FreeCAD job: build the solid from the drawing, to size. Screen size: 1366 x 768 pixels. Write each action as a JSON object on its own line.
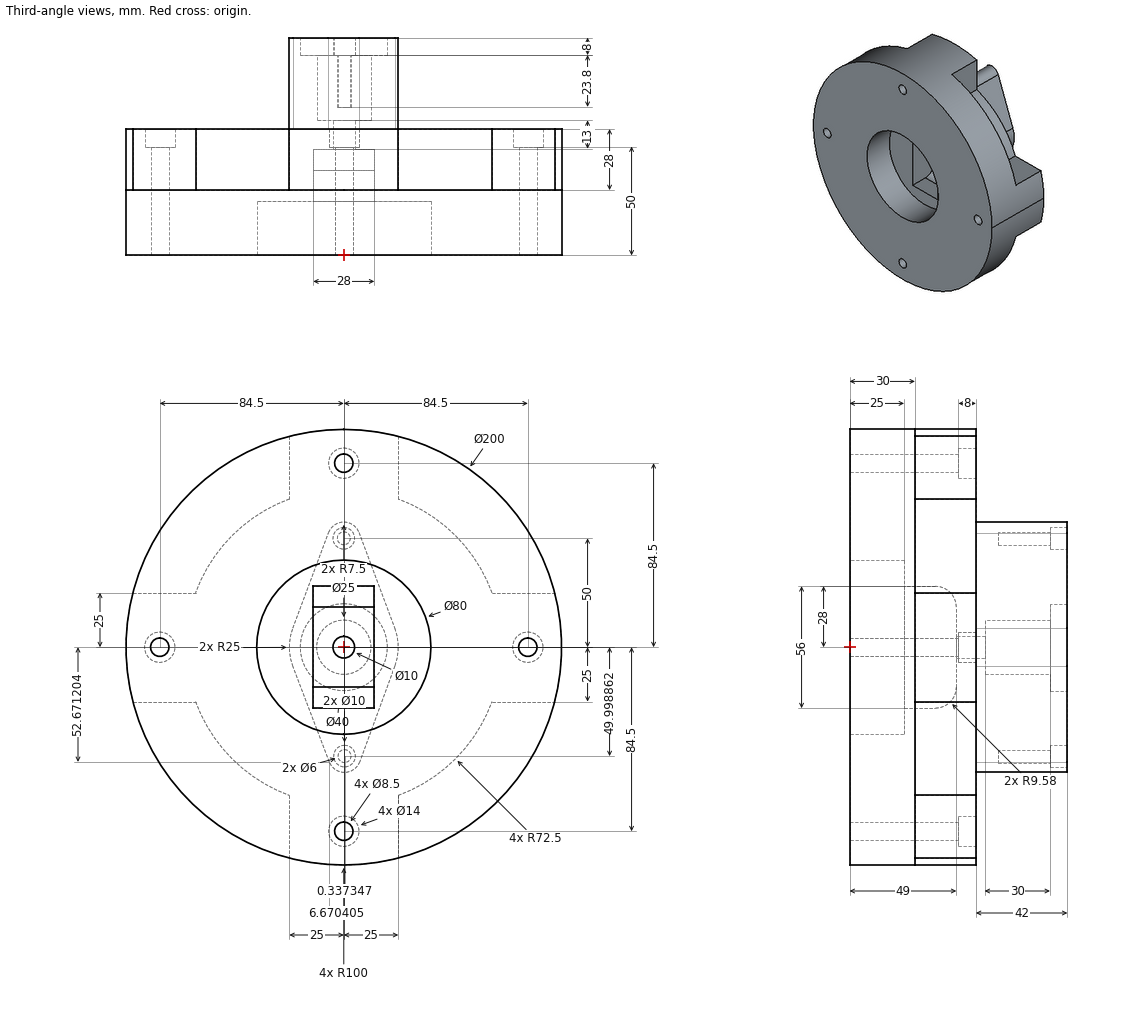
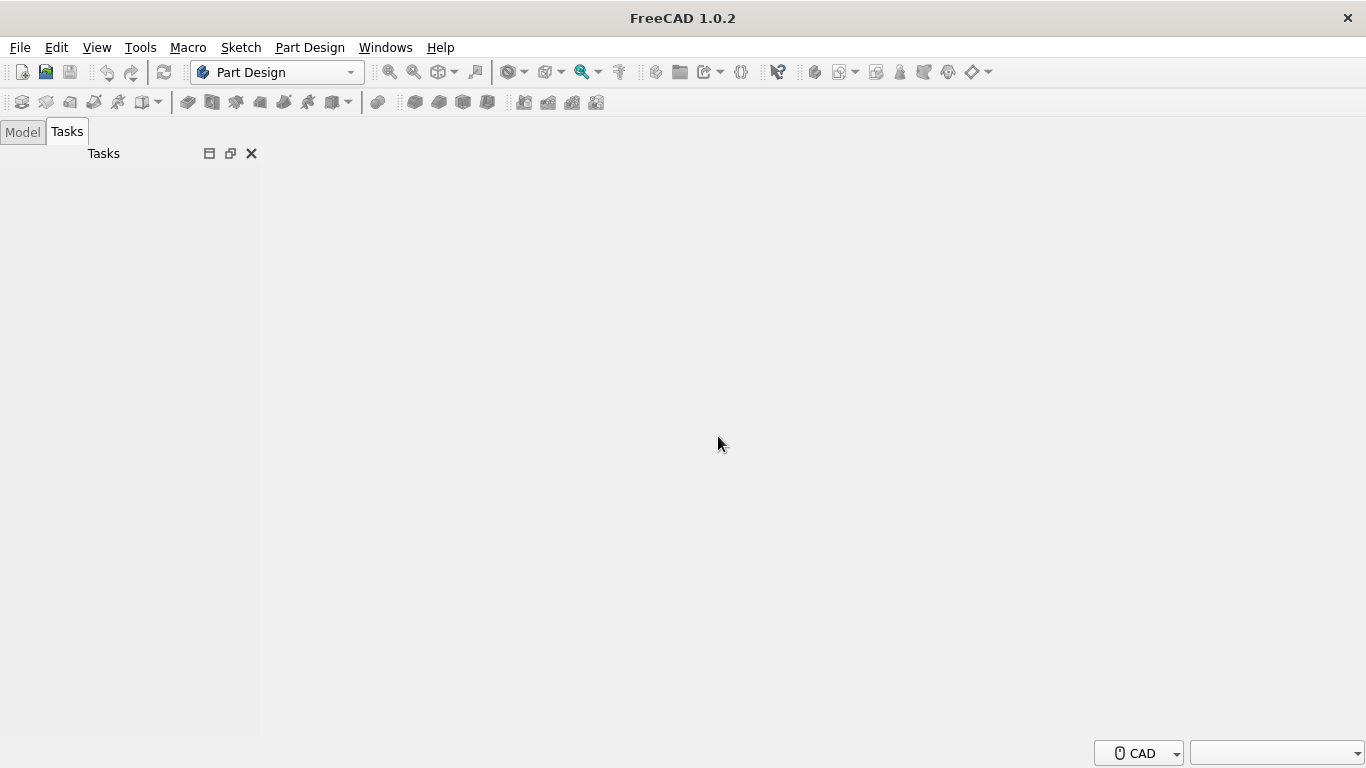
{"action": "key", "text": "ctrl+n"}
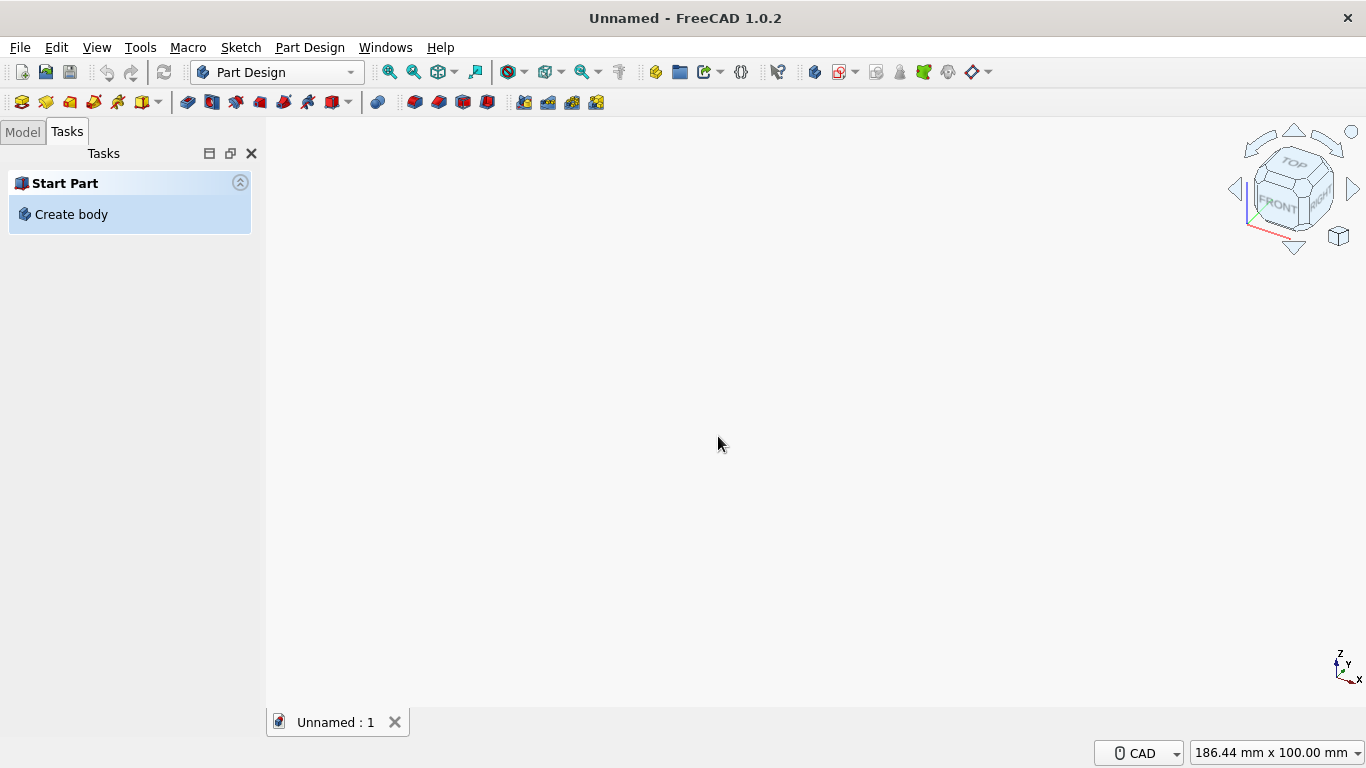
{"action": "left_click", "coordinate": [840, 72]}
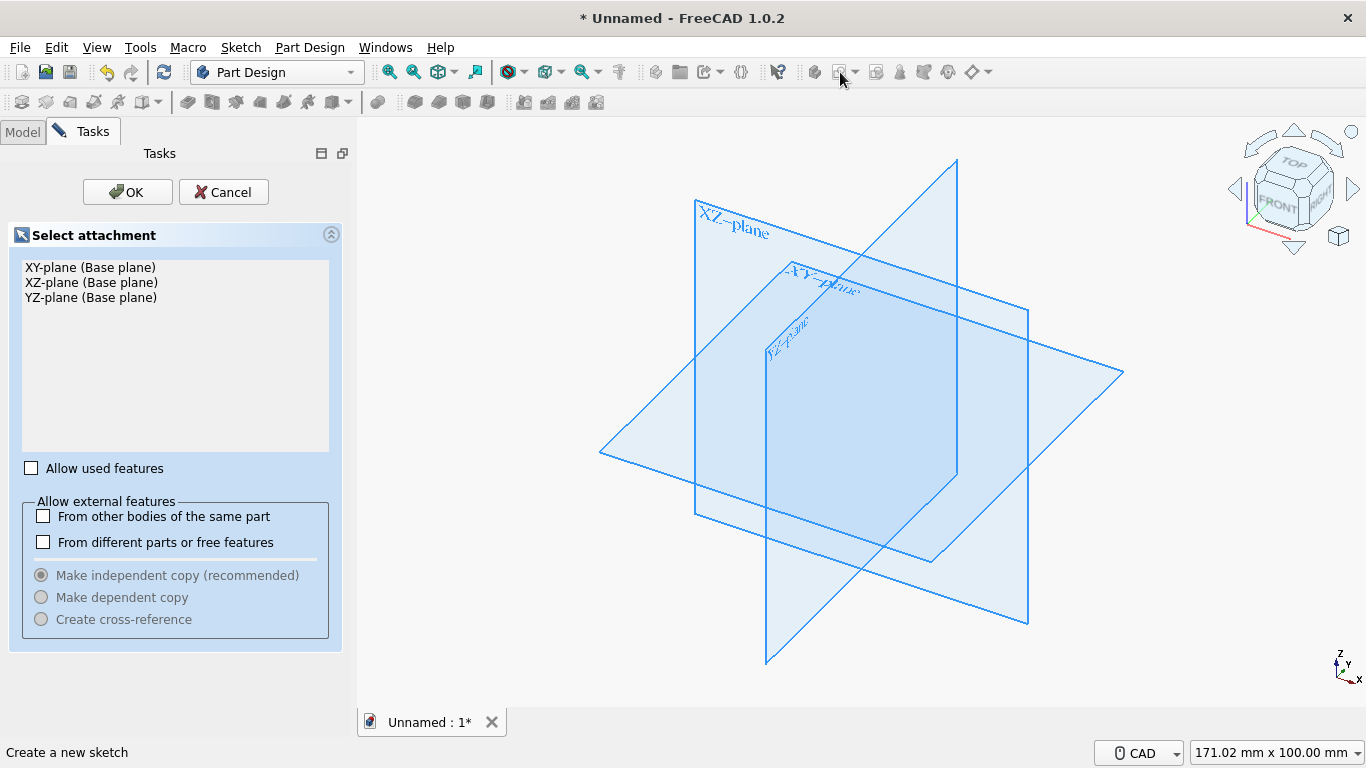
{"action": "left_click", "coordinate": [82, 282]}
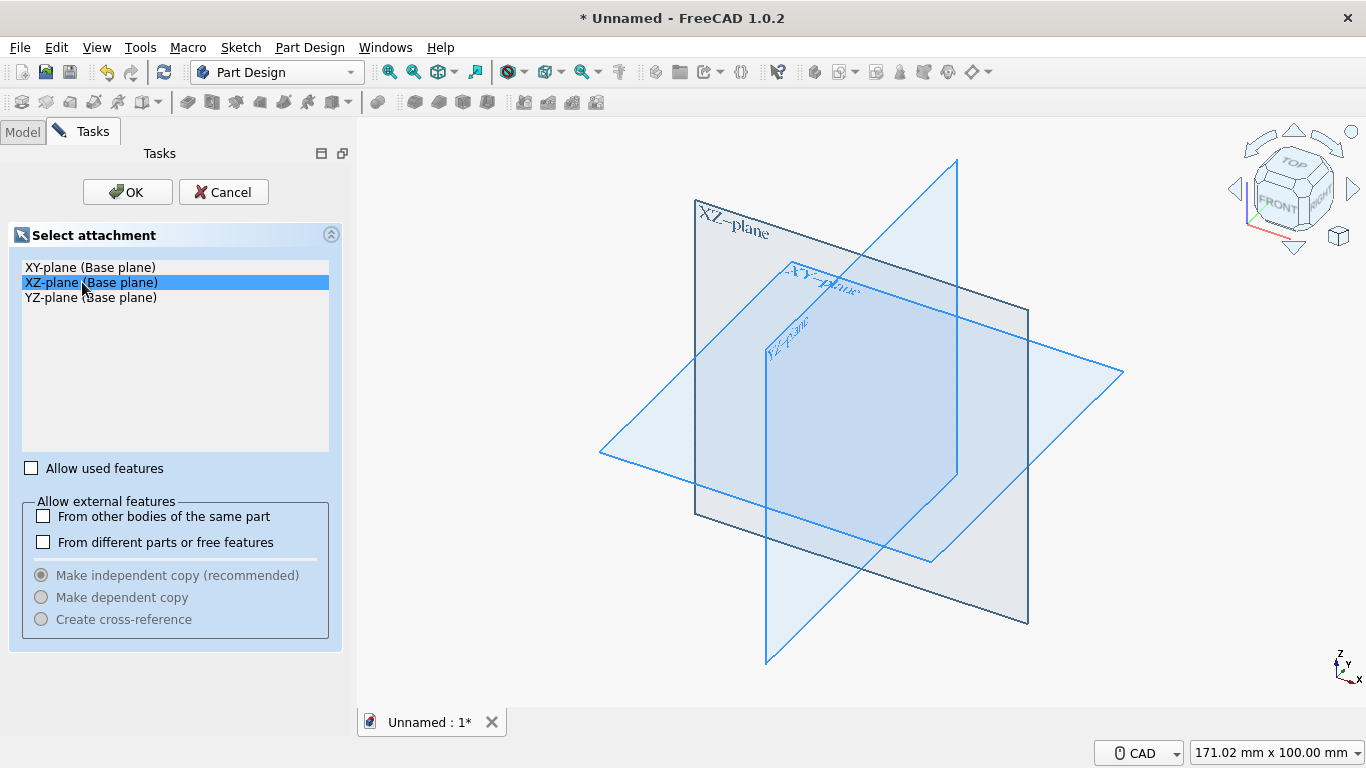
{"action": "left_click", "coordinate": [128, 192]}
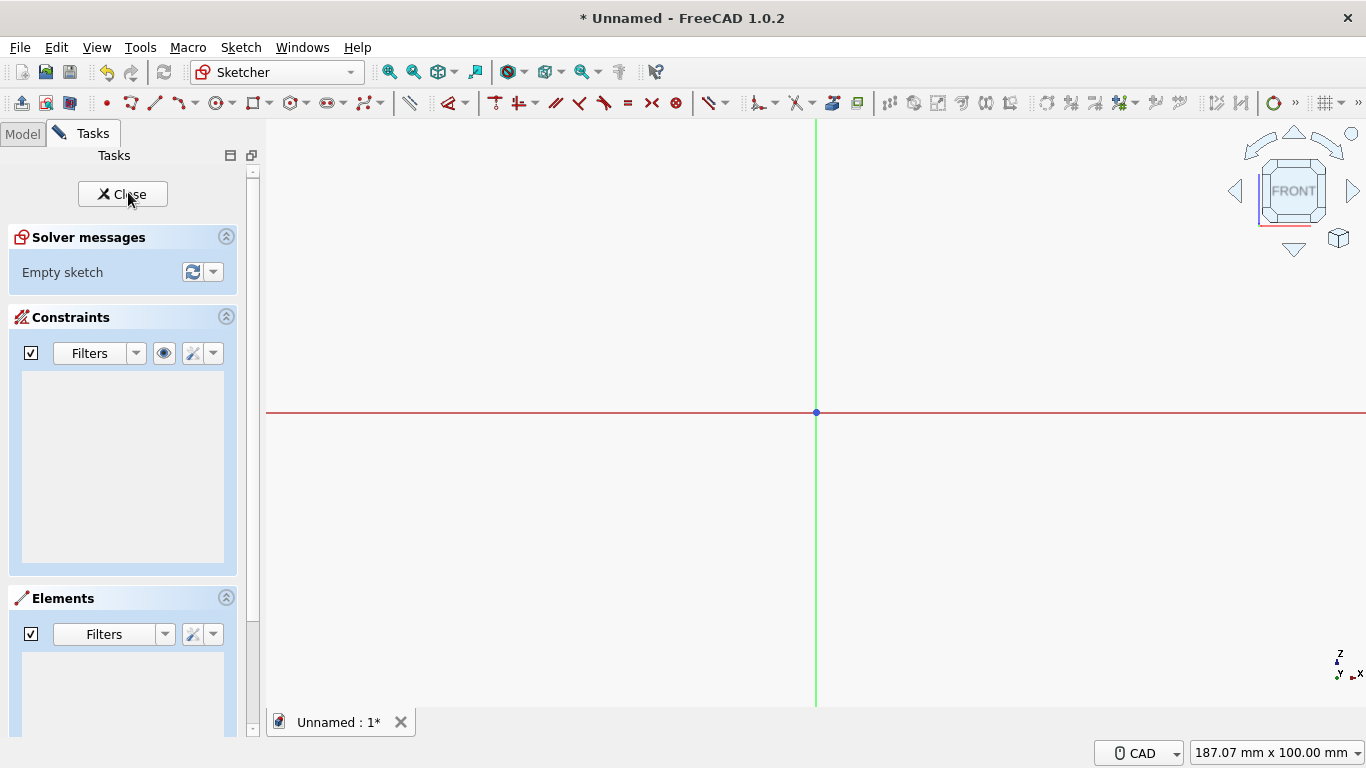
{"action": "scroll", "coordinate": [718, 413], "scroll_direction": "down", "scroll_amount": 6}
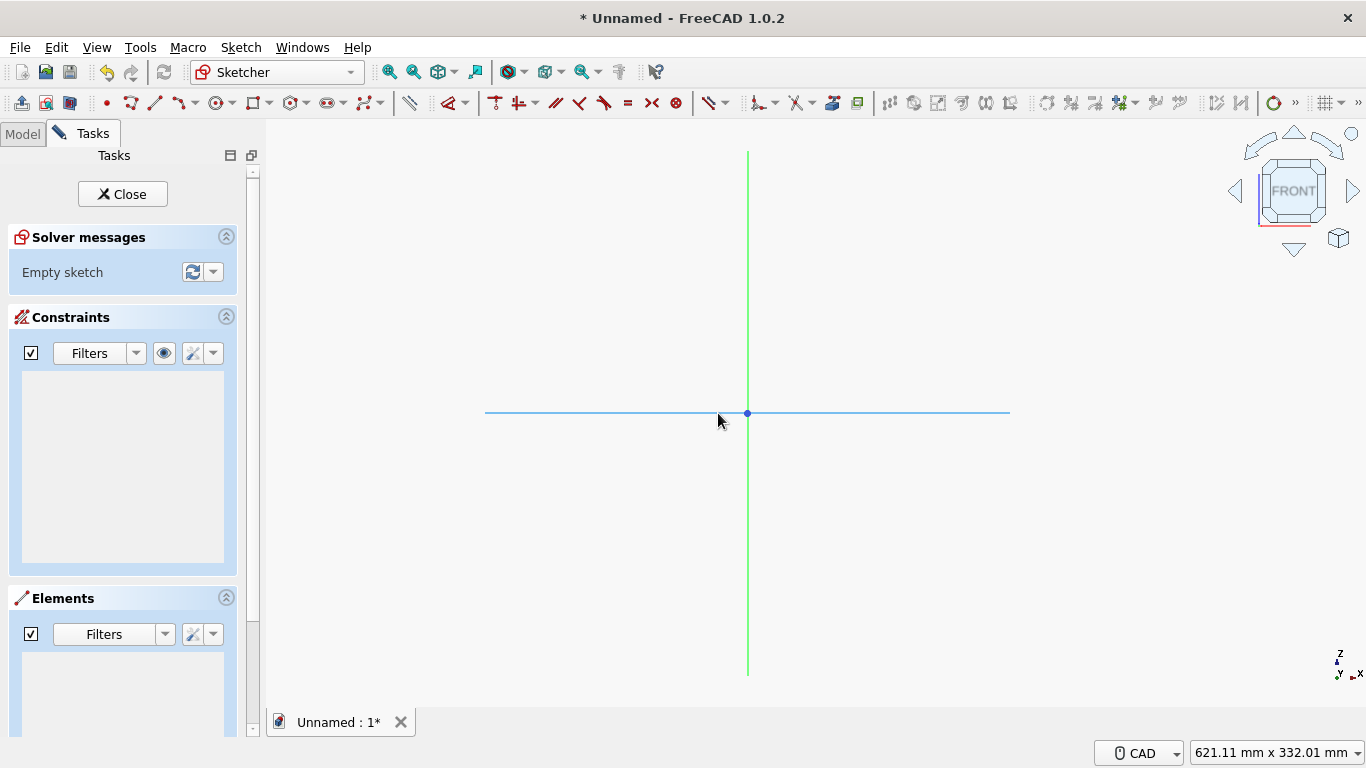
{"action": "key", "text": "g c"}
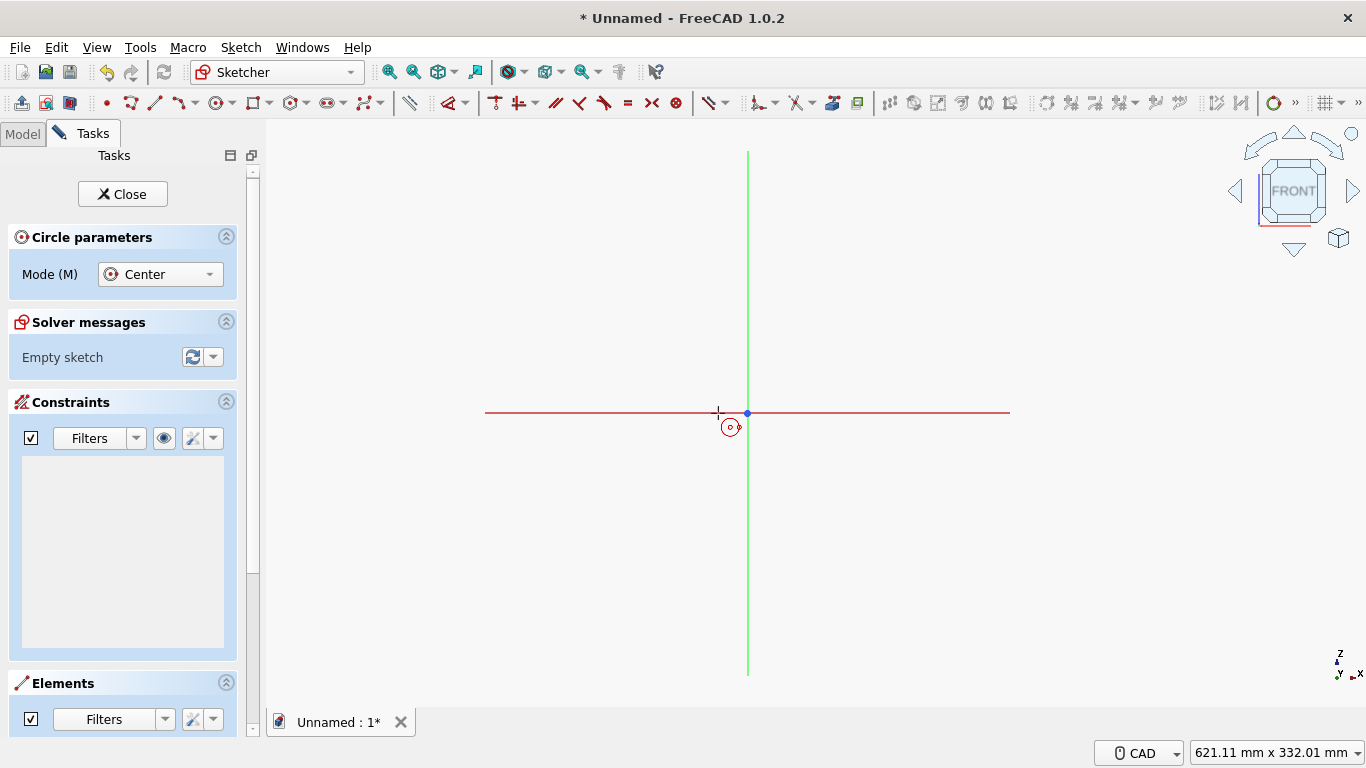
{"action": "left_click", "coordinate": [748, 413]}
{"action": "left_click", "coordinate": [873, 288]}
{"action": "key", "text": "Escape"}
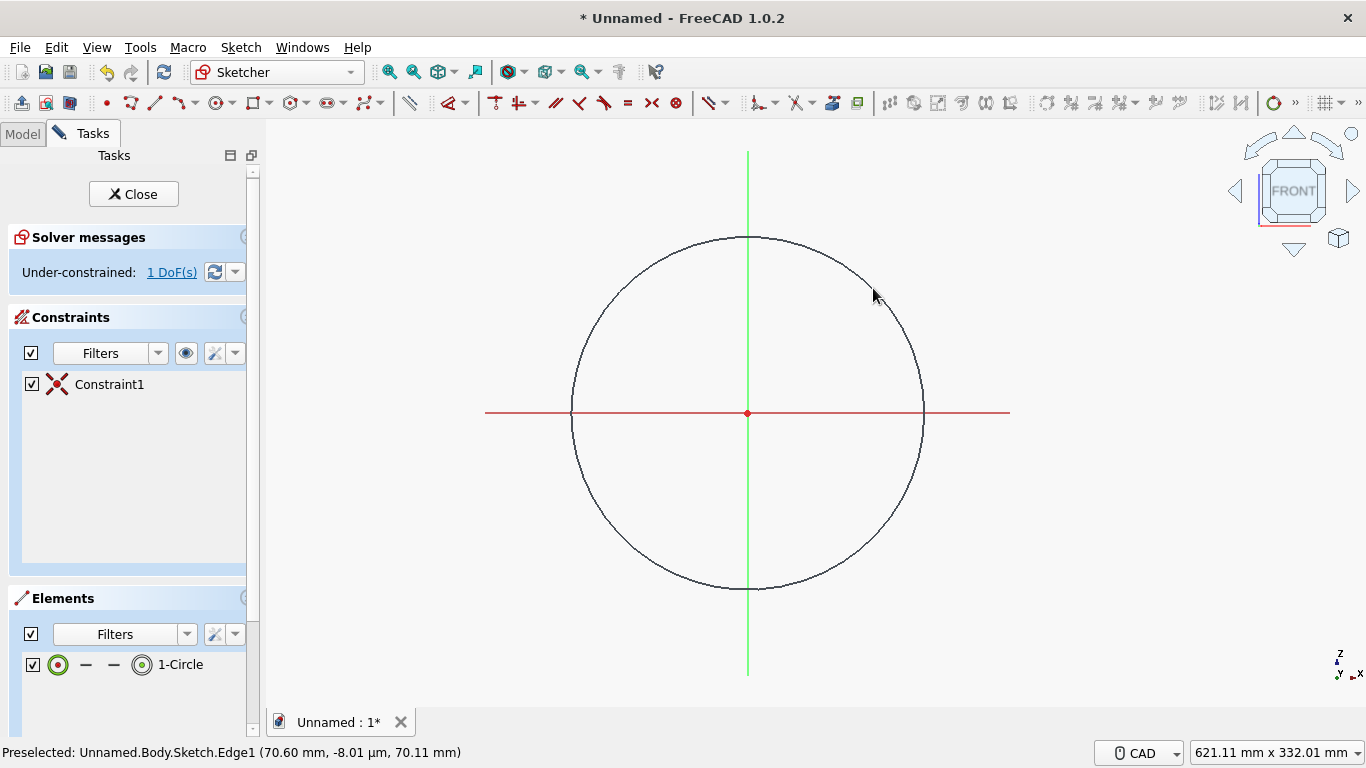
{"action": "key", "text": "d"}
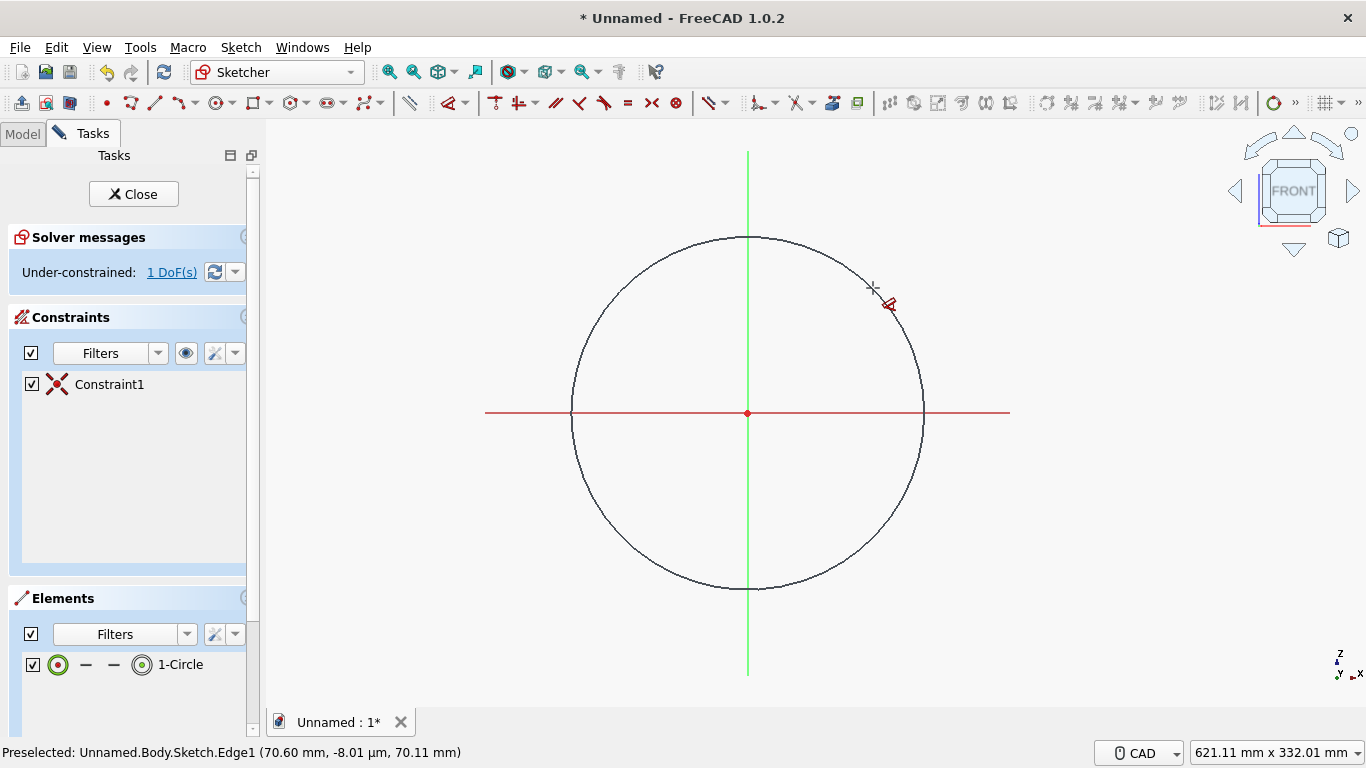
{"action": "left_click", "coordinate": [872, 288]}
{"action": "left_click", "coordinate": [895, 265]}